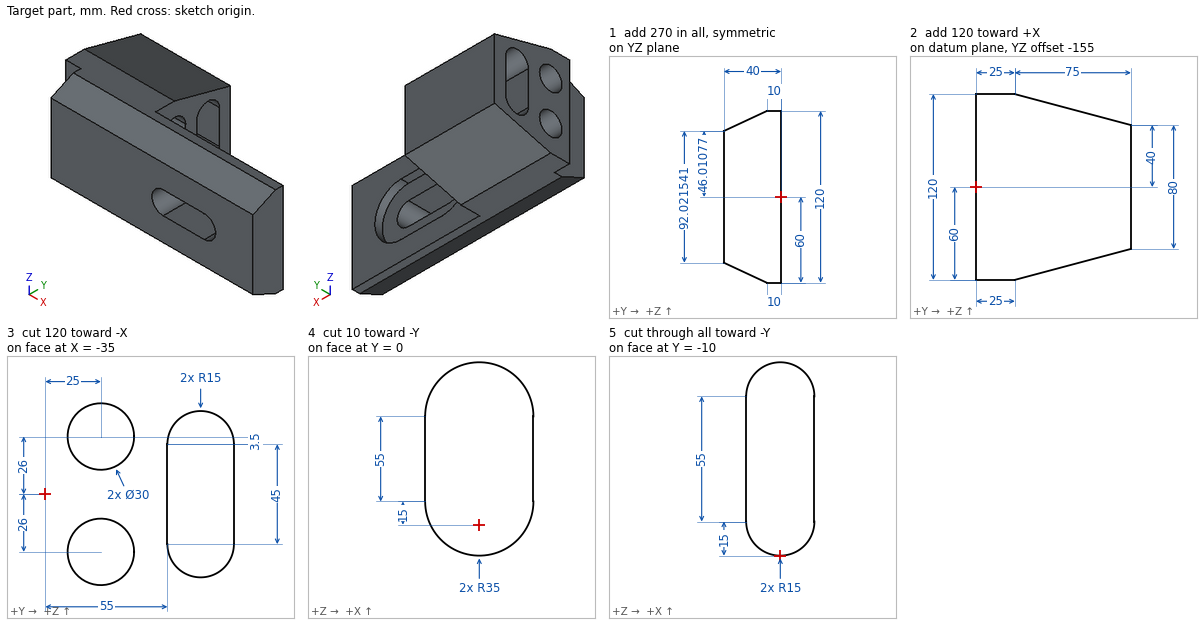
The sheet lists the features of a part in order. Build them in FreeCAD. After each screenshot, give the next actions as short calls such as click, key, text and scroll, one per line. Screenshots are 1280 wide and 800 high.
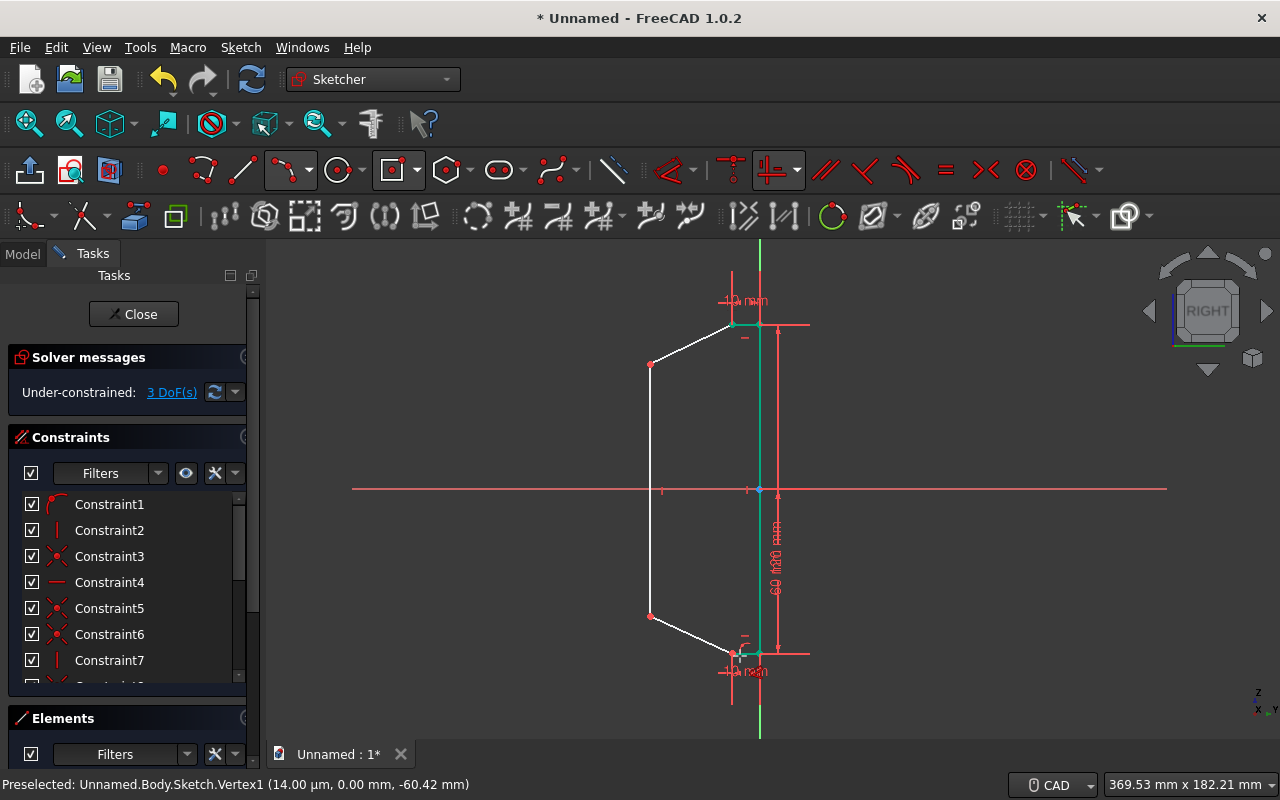
click(650, 364)
click(680, 330)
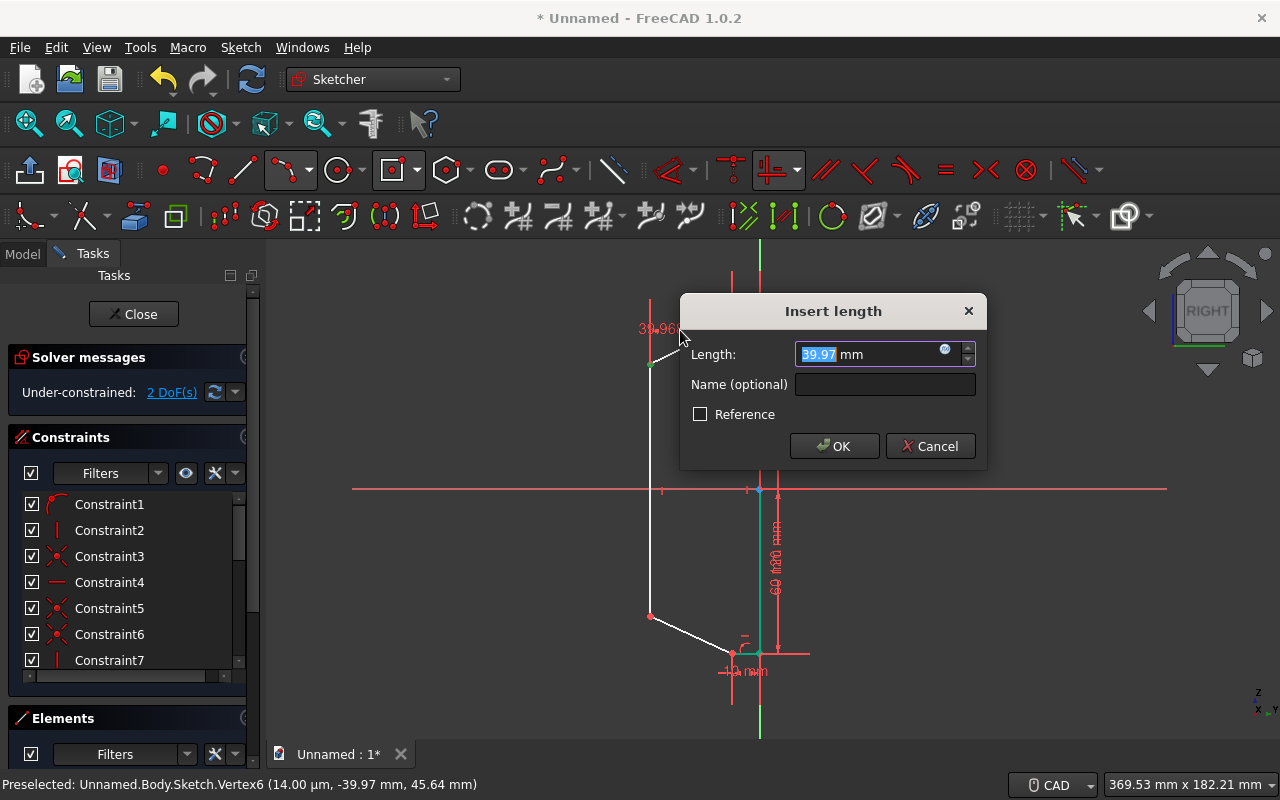
text(40)
key(Return)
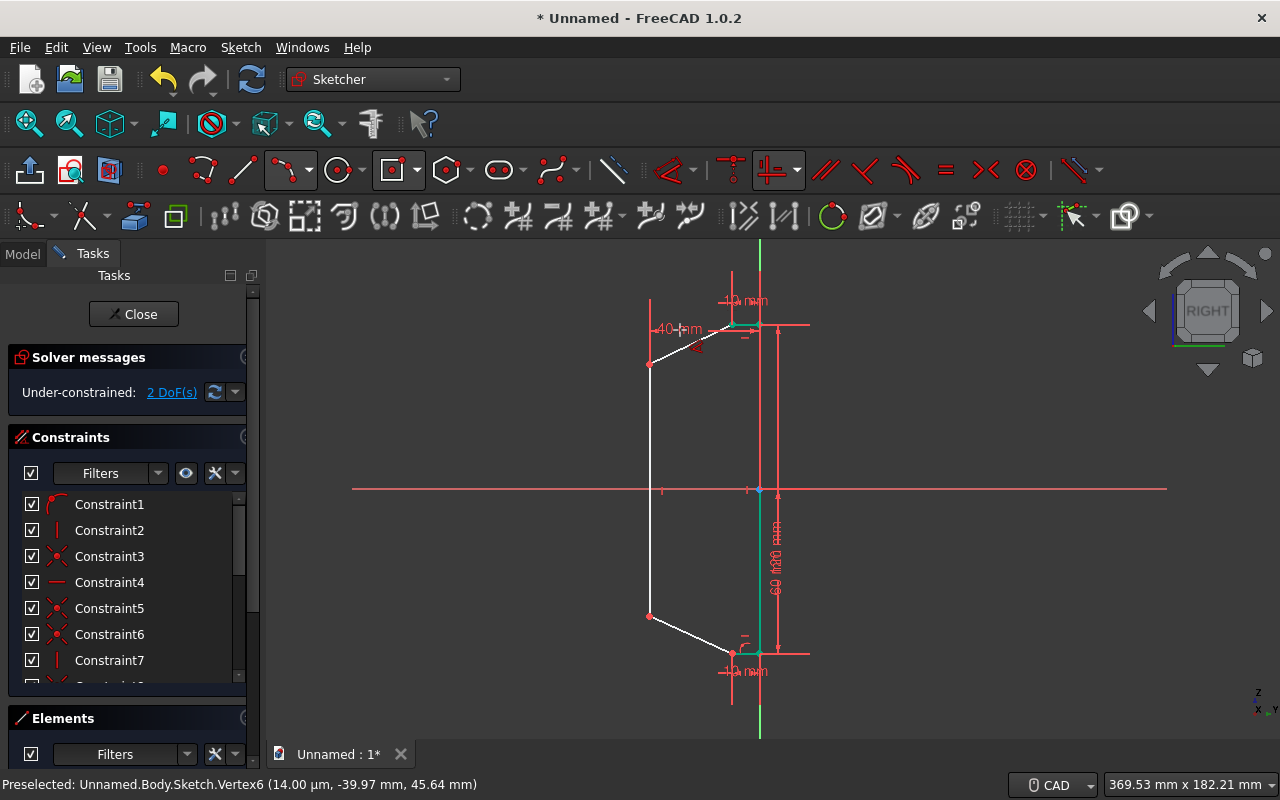
click(650, 440)
click(616, 432)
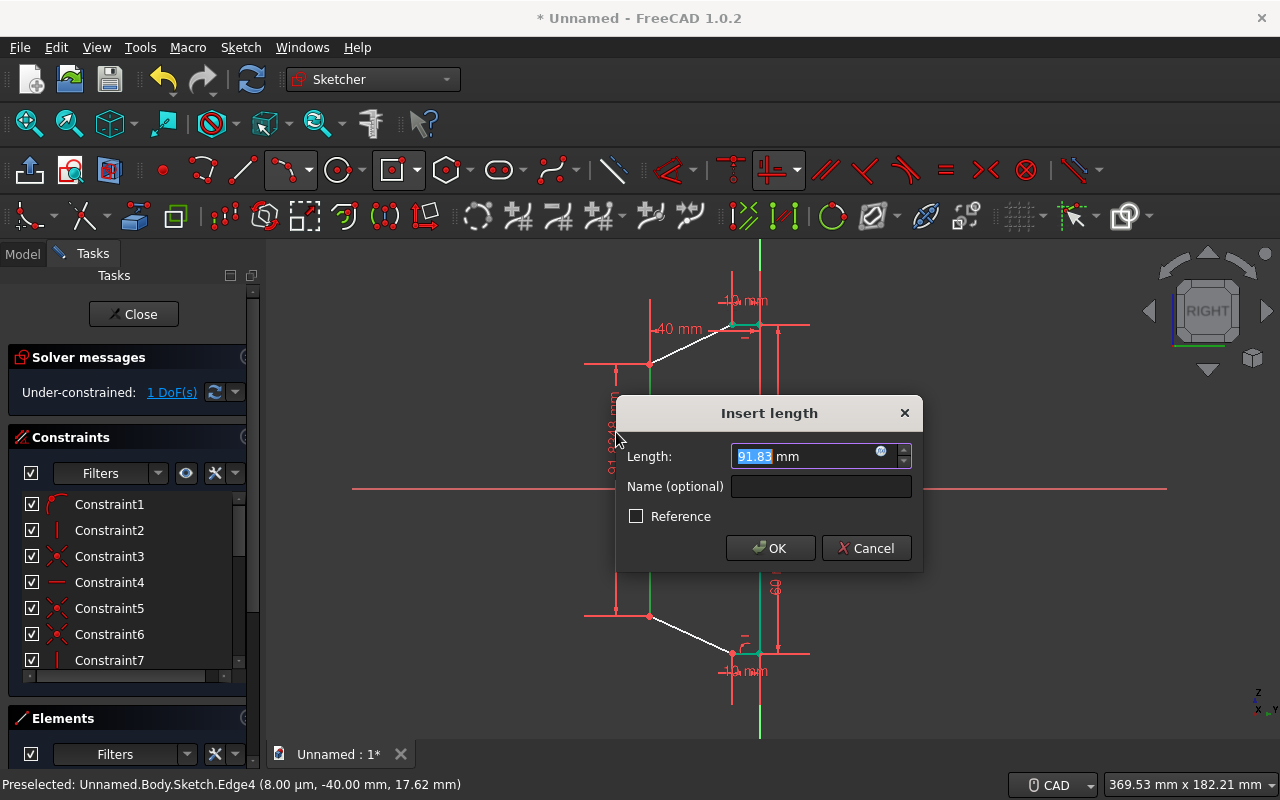
text(92.021541)
key(Return)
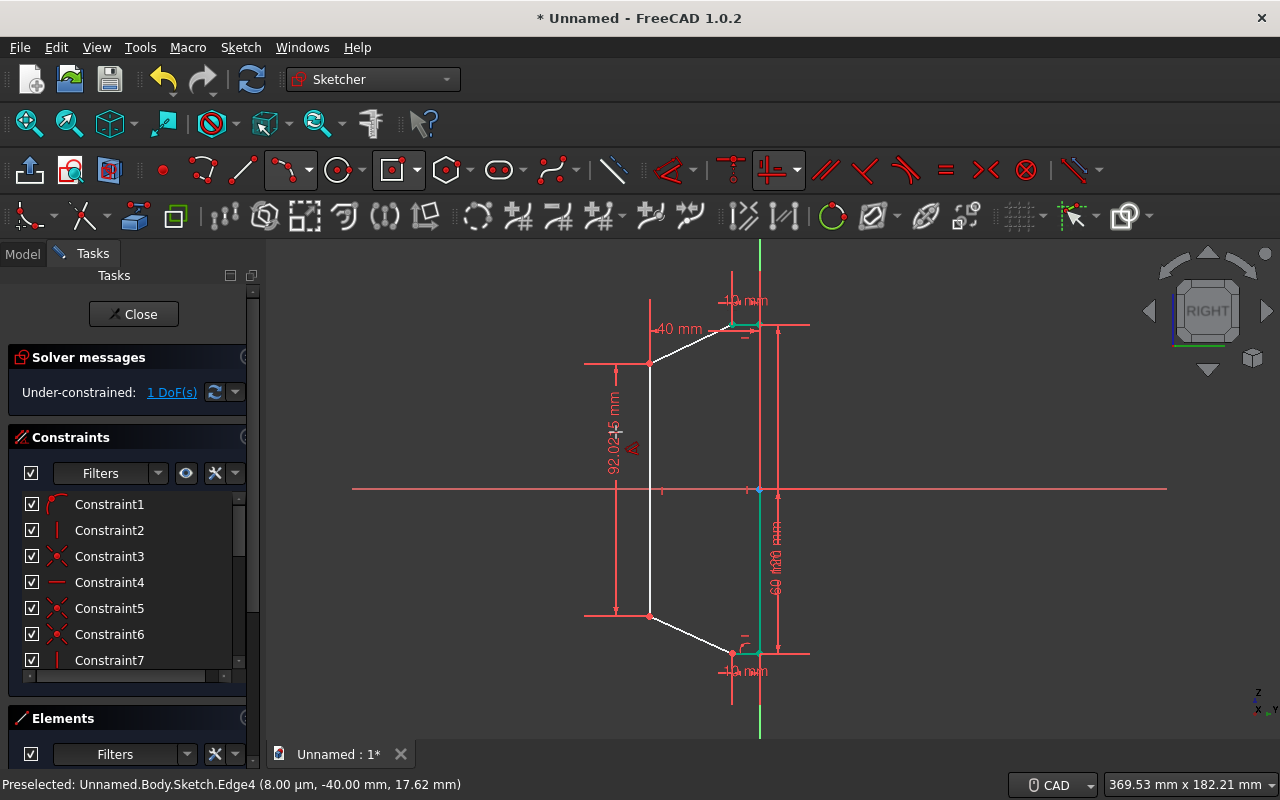
click(650, 364)
click(794, 427)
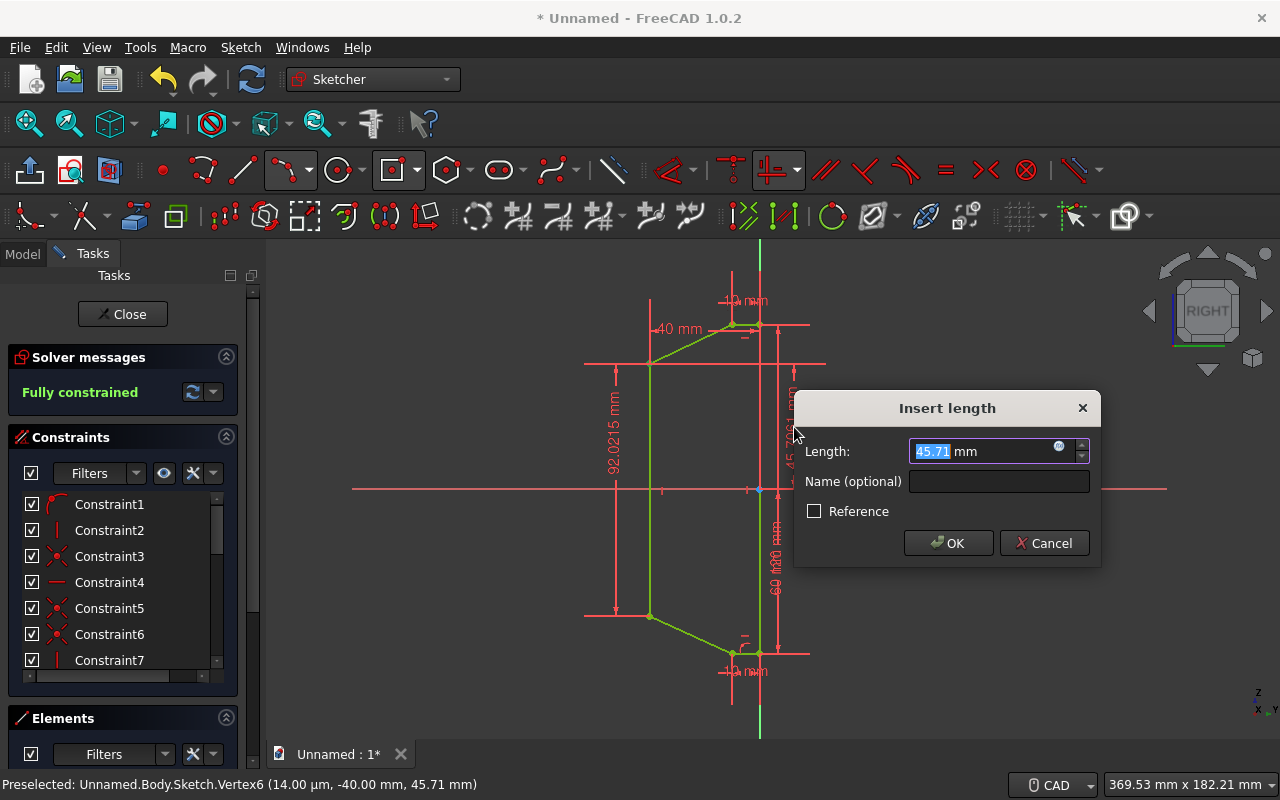
text(46.01077)
key(Return)
key(Escape)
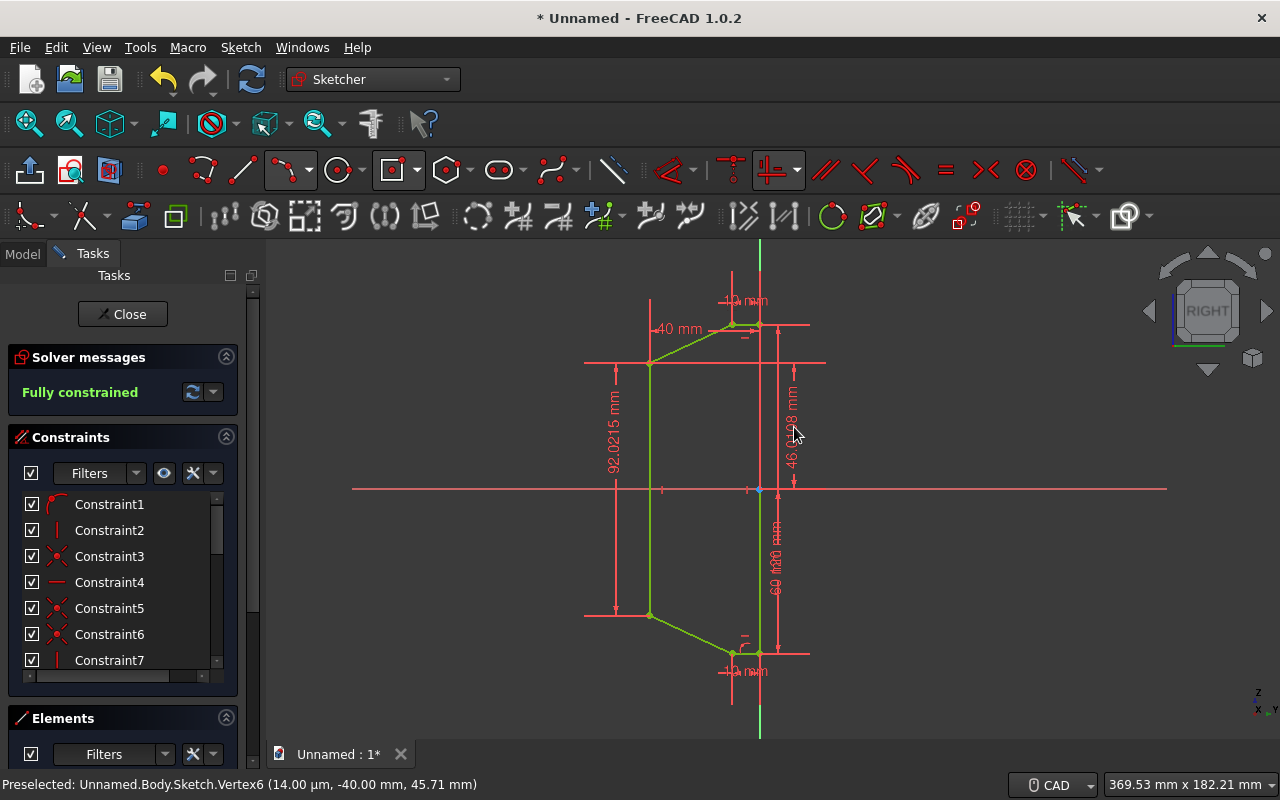
click(123, 314)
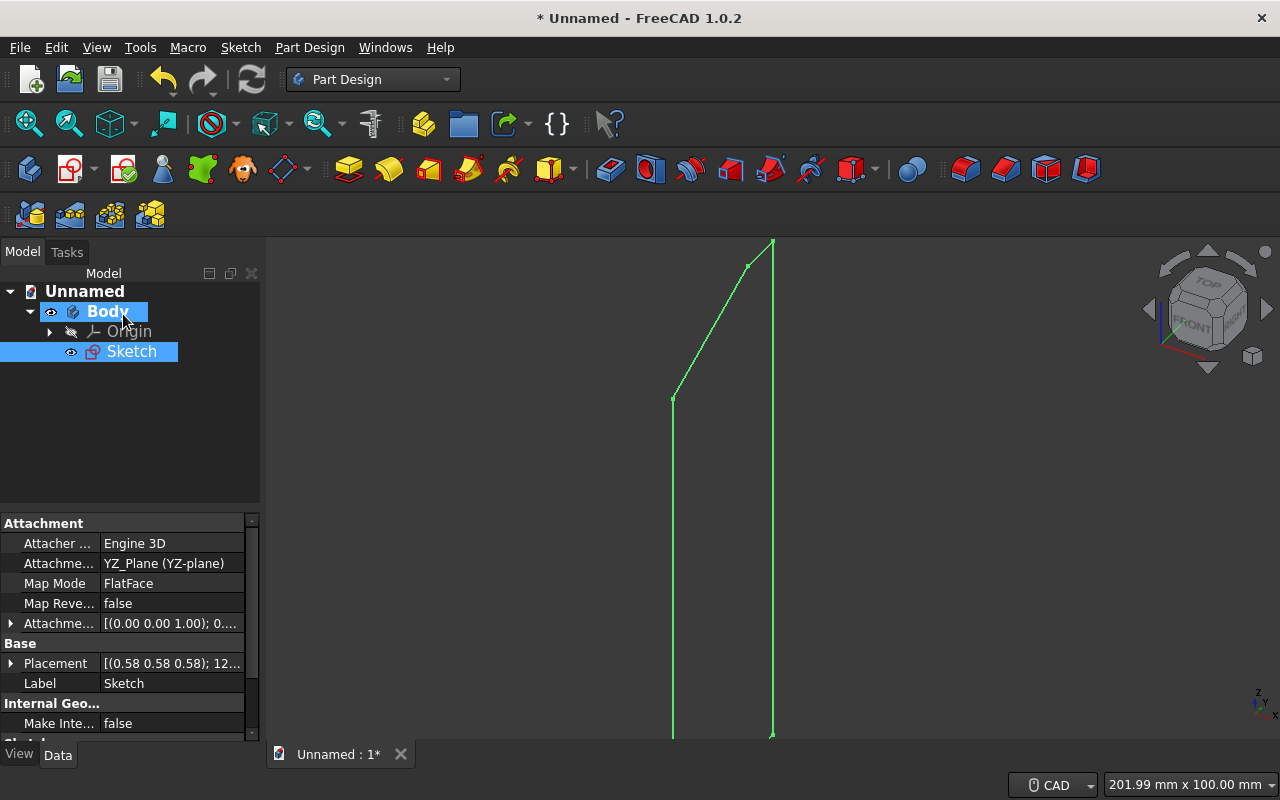
click(350, 170)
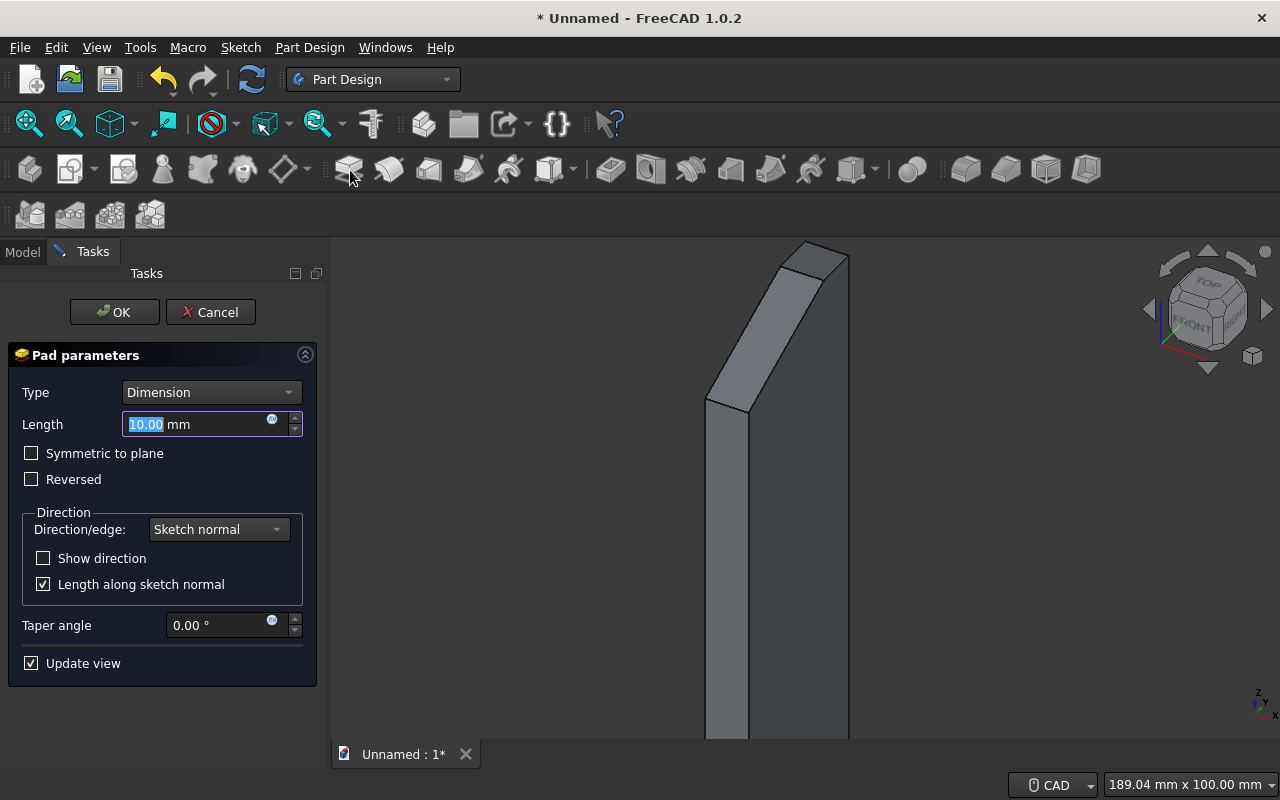
text(270)
key(Tab)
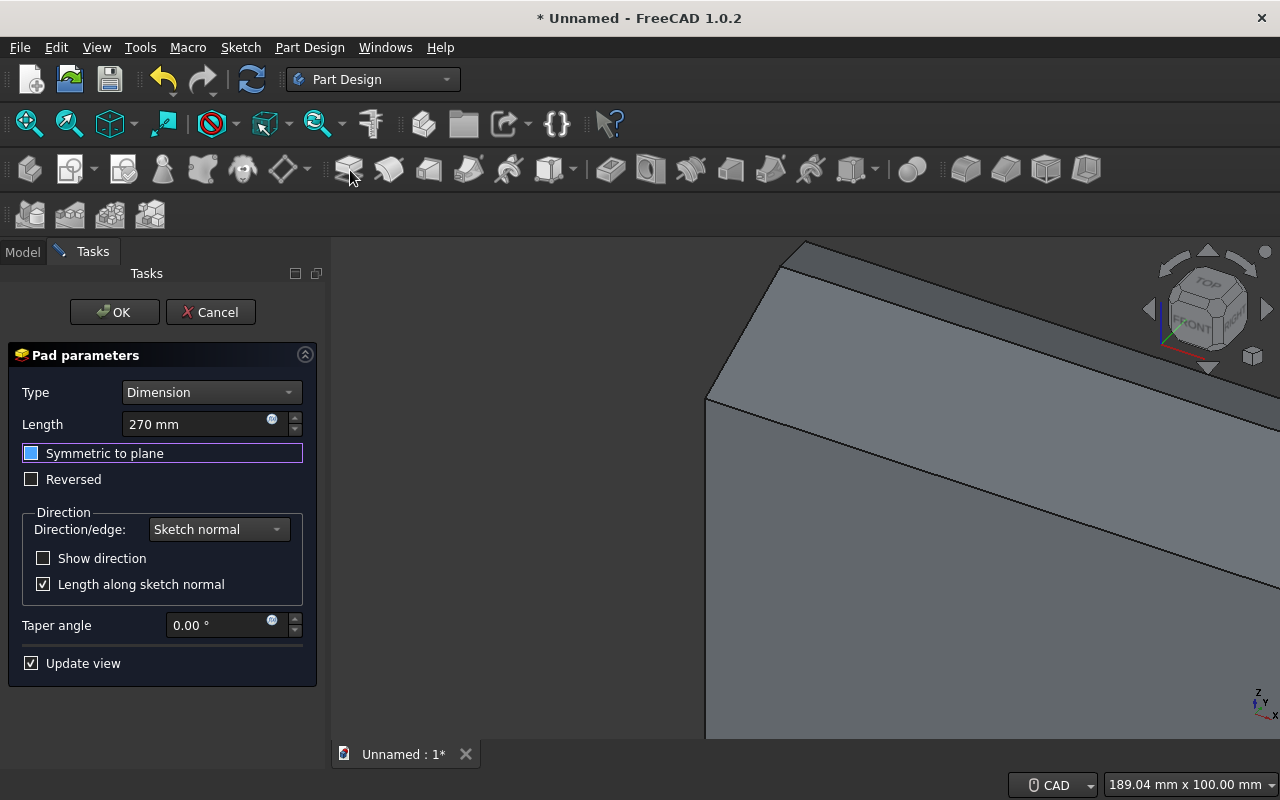
click(30, 453)